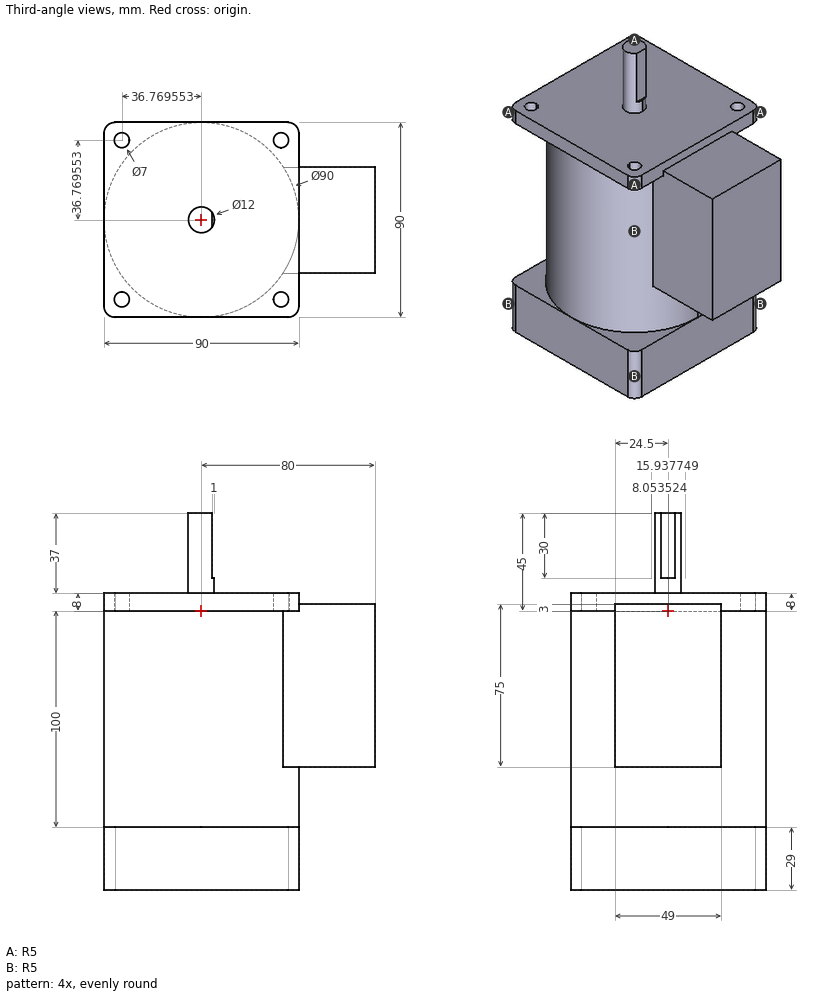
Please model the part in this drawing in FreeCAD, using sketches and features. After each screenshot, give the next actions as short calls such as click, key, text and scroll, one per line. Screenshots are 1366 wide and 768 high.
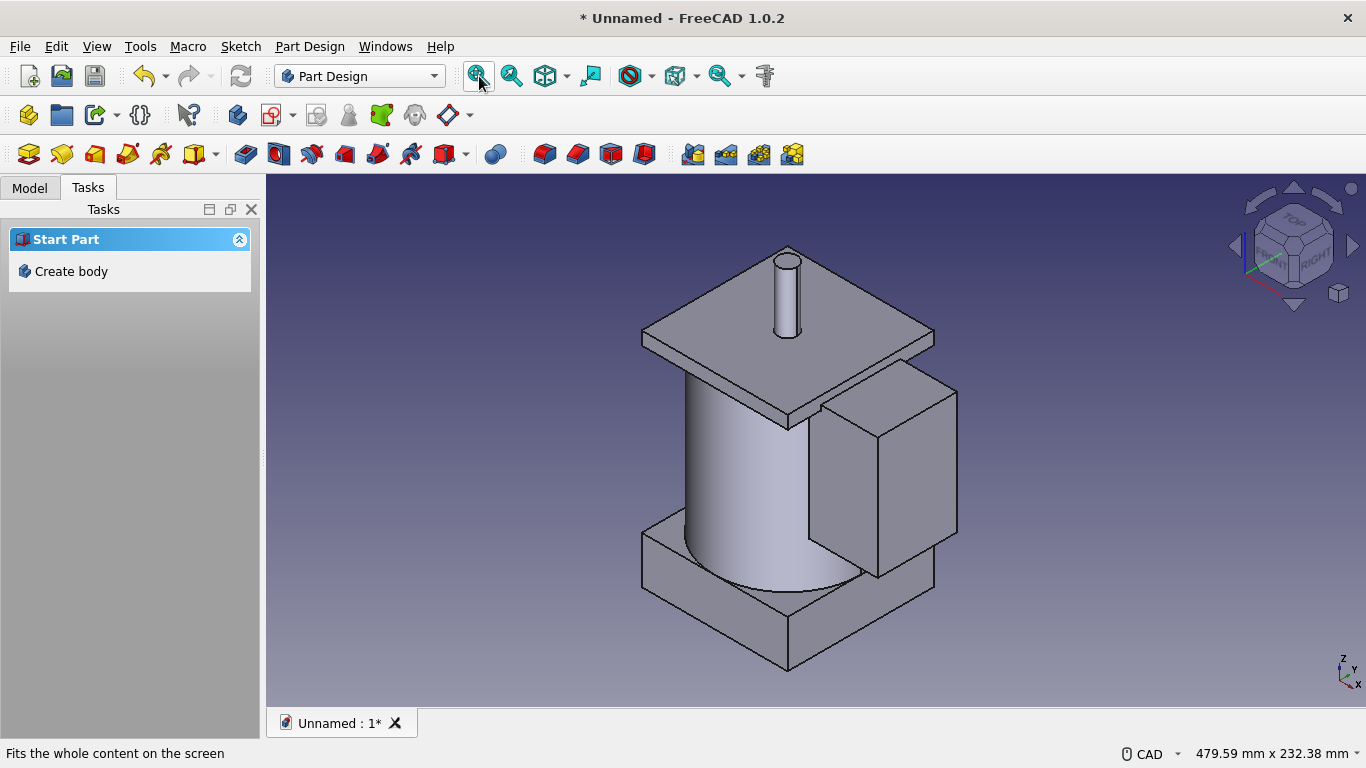
click(871, 329)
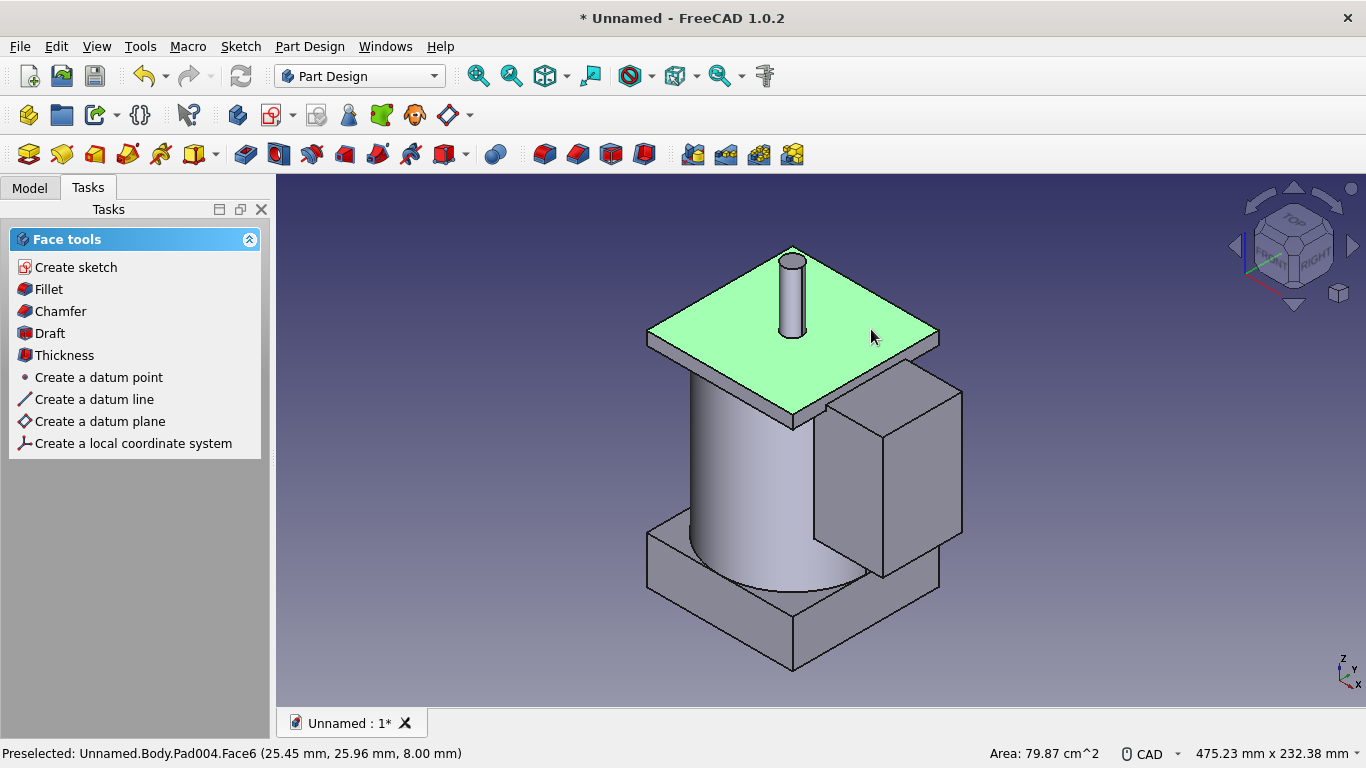
click(270, 116)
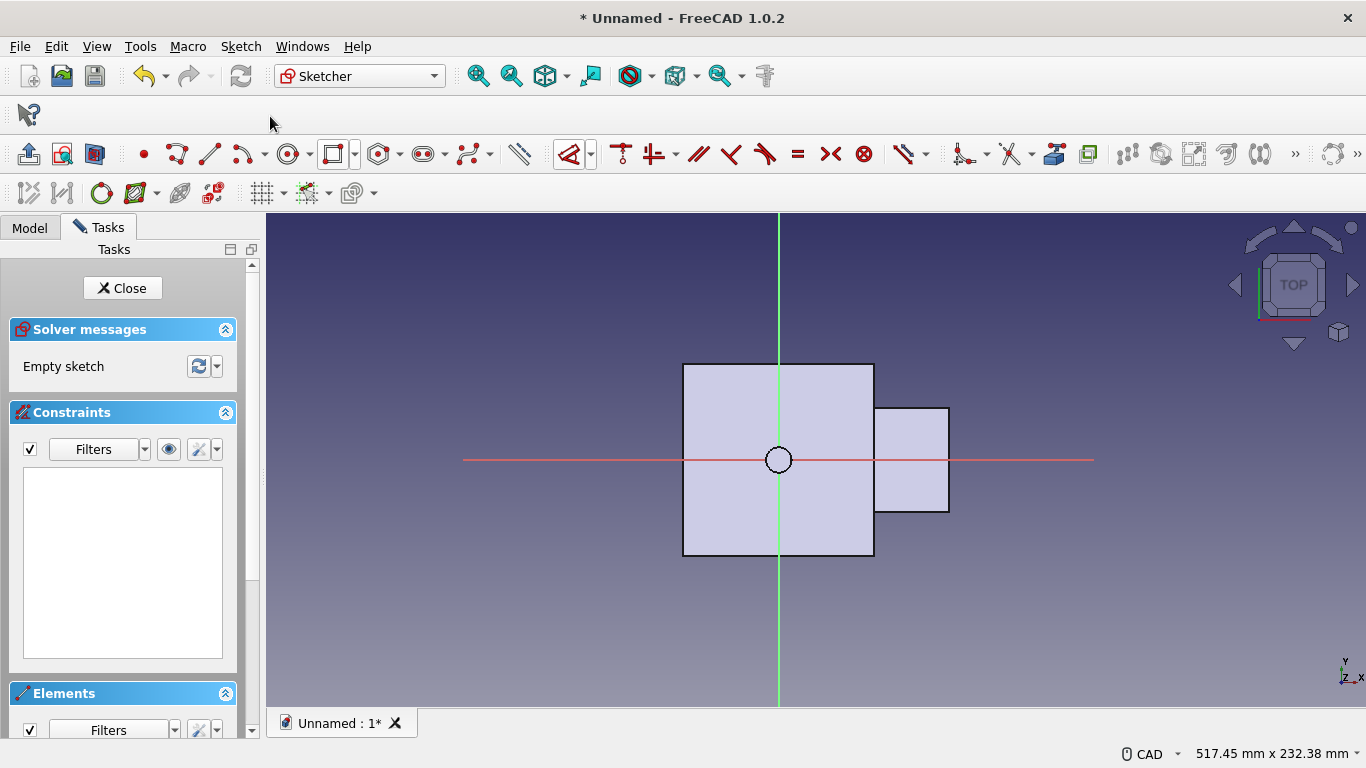
click(95, 154)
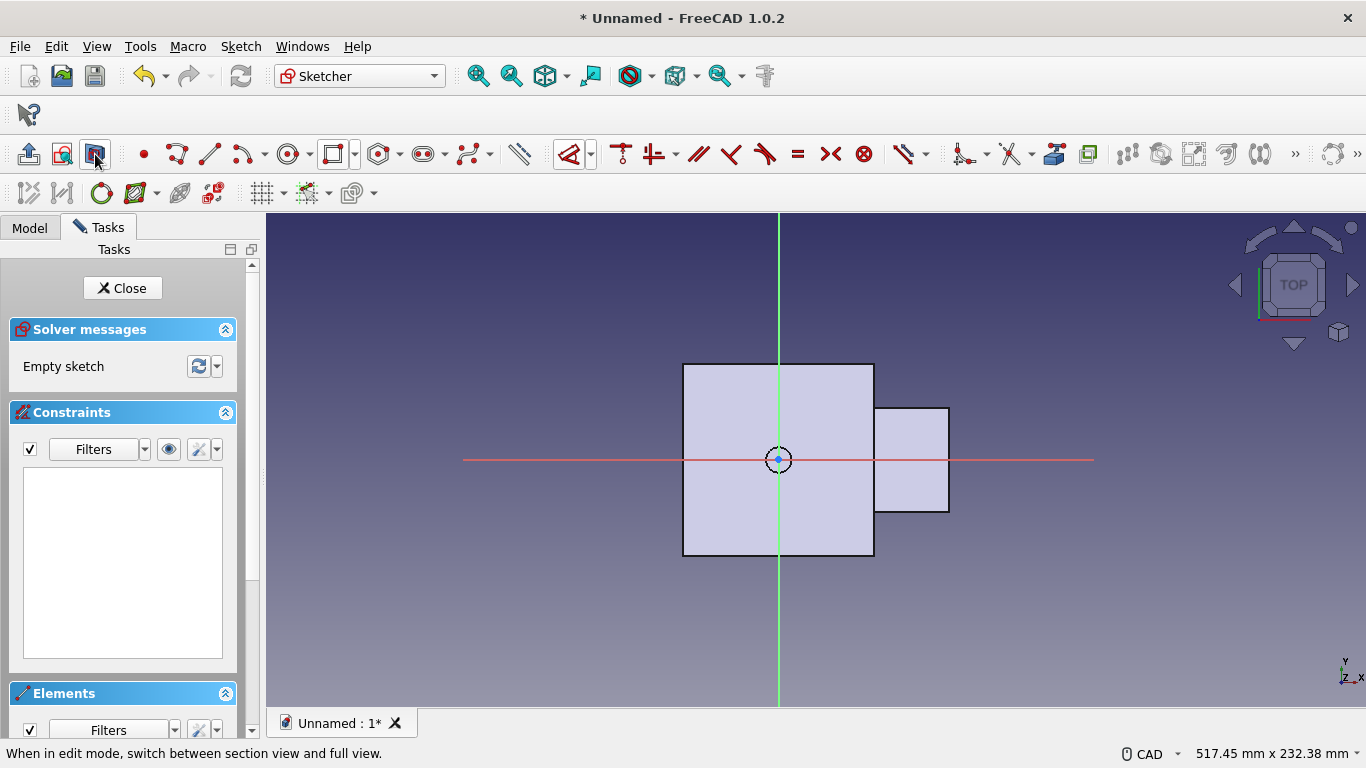
scroll(698, 378, up, 15)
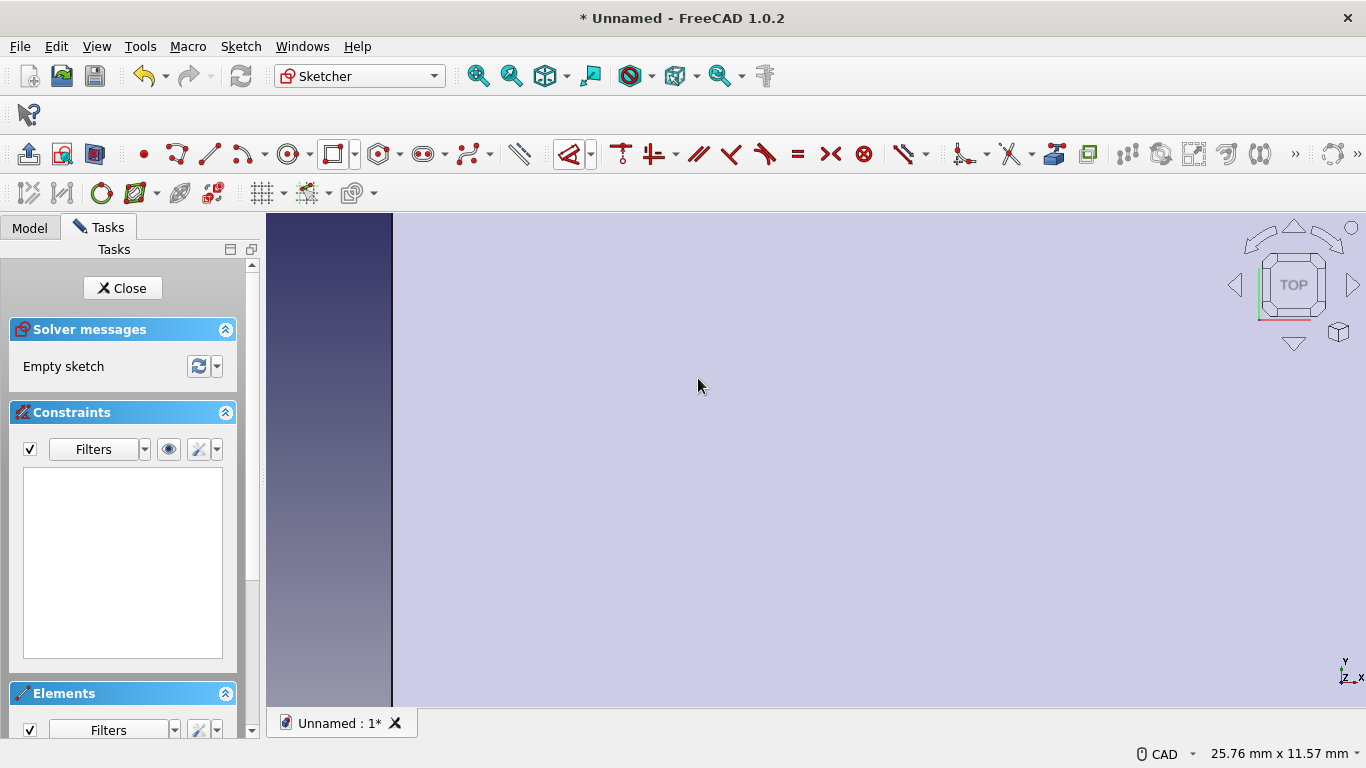
click(288, 154)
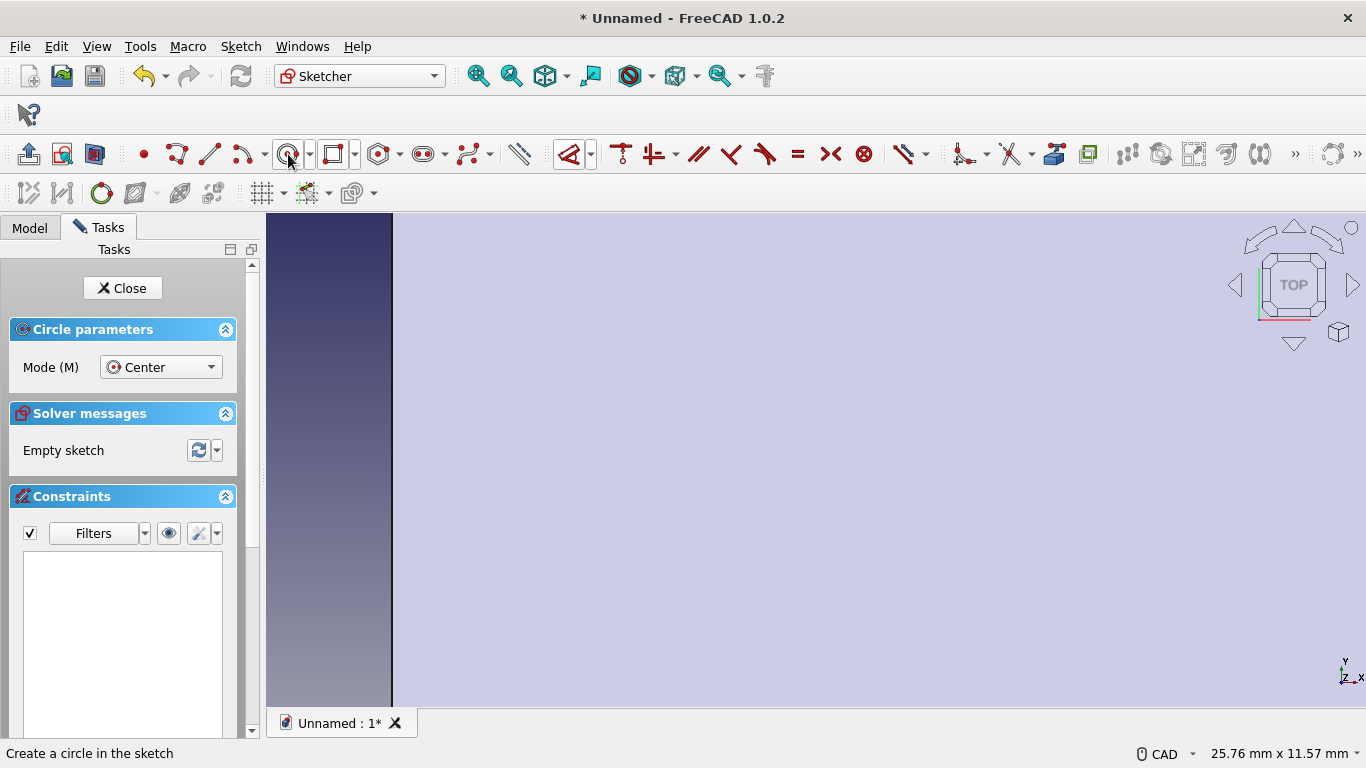
click(743, 449)
click(849, 343)
key(Escape)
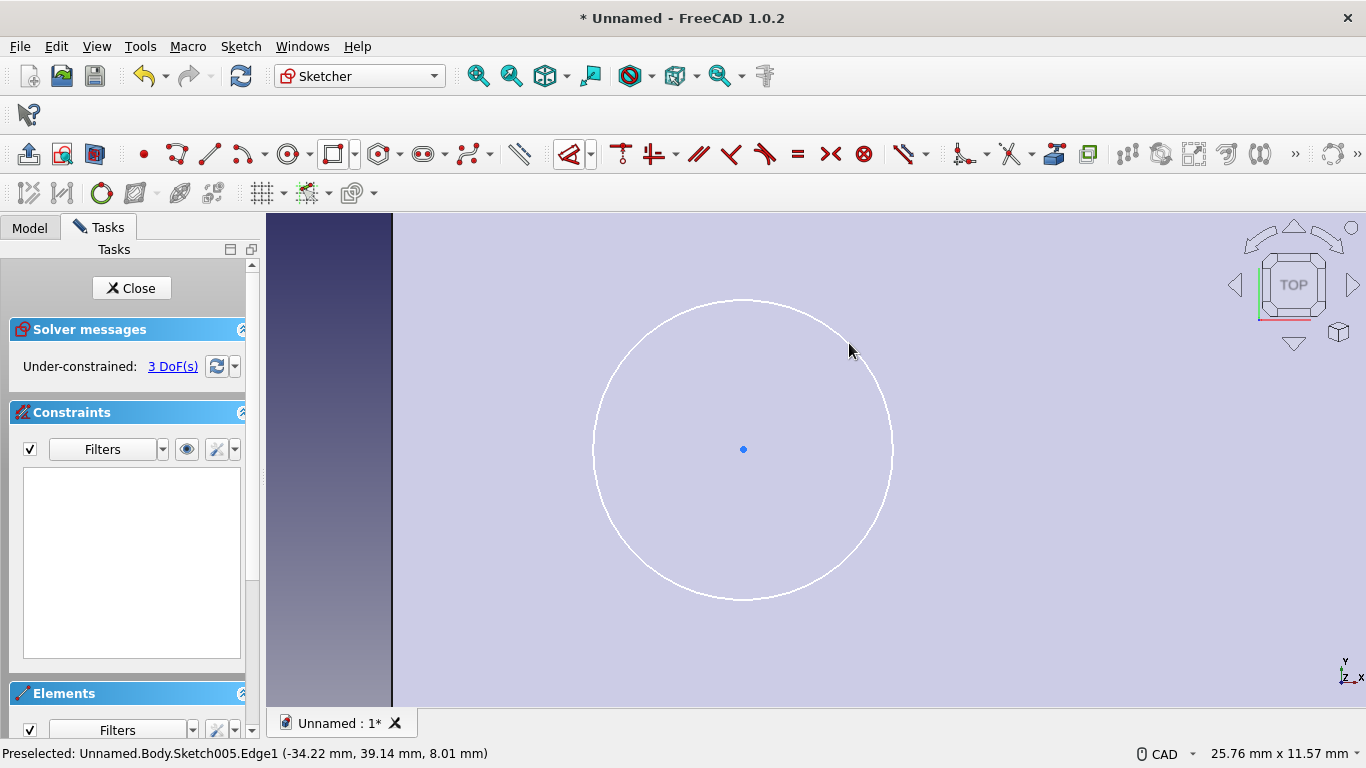
click(849, 344)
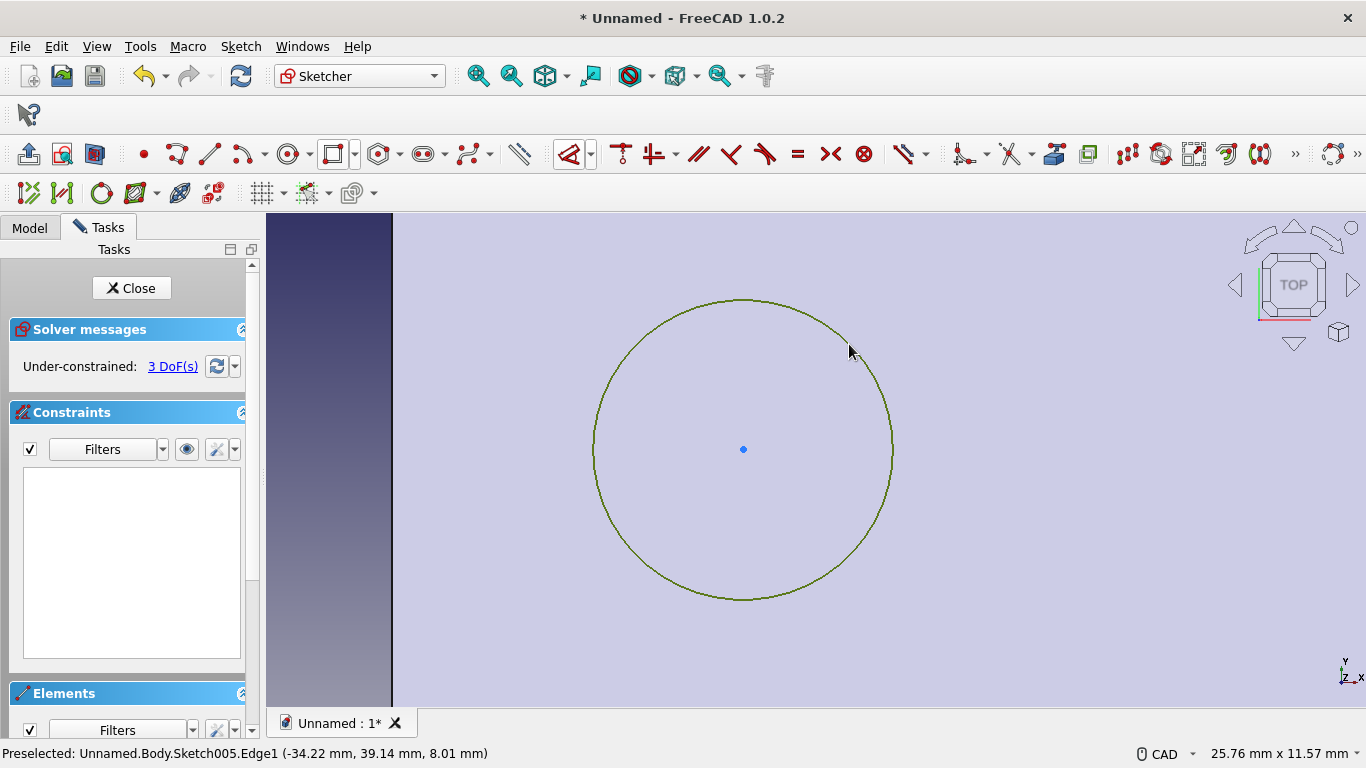
key(k)
key(o)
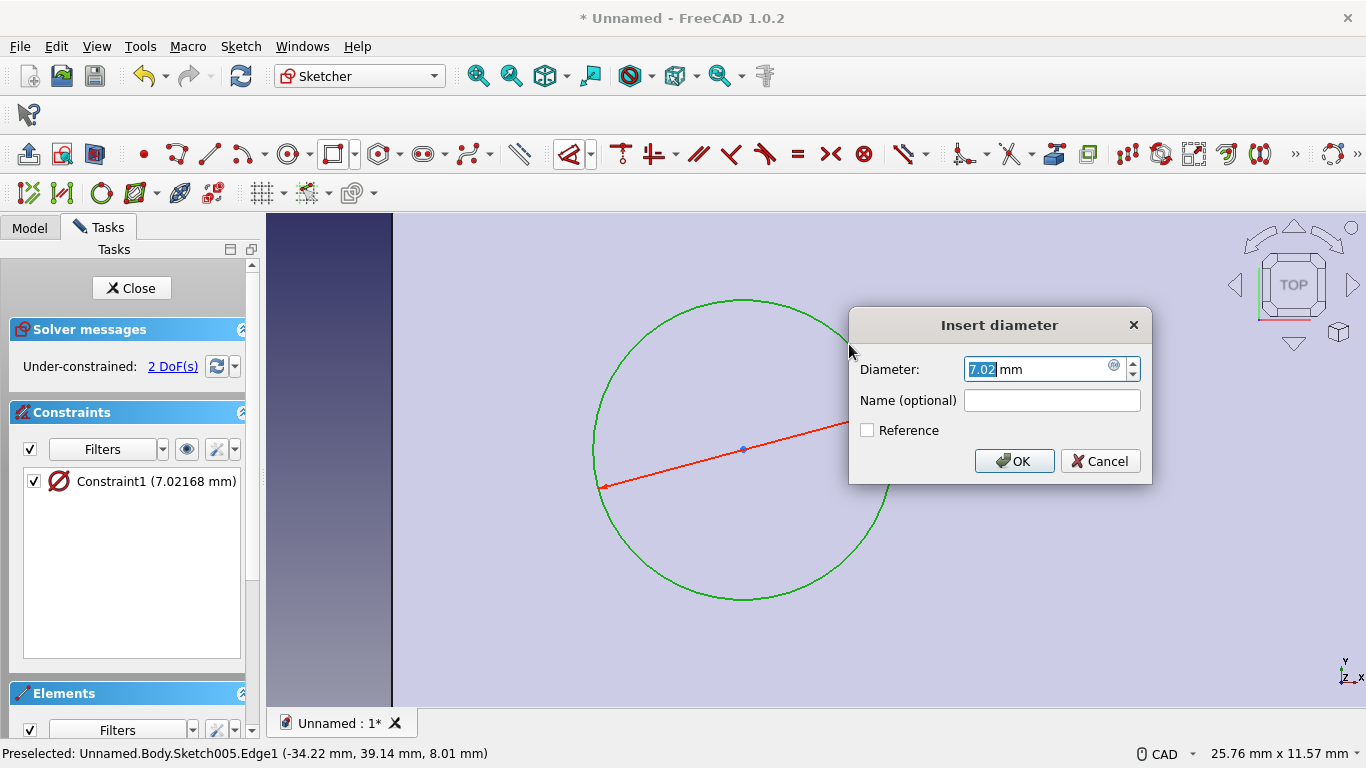
text(7)
key(Return)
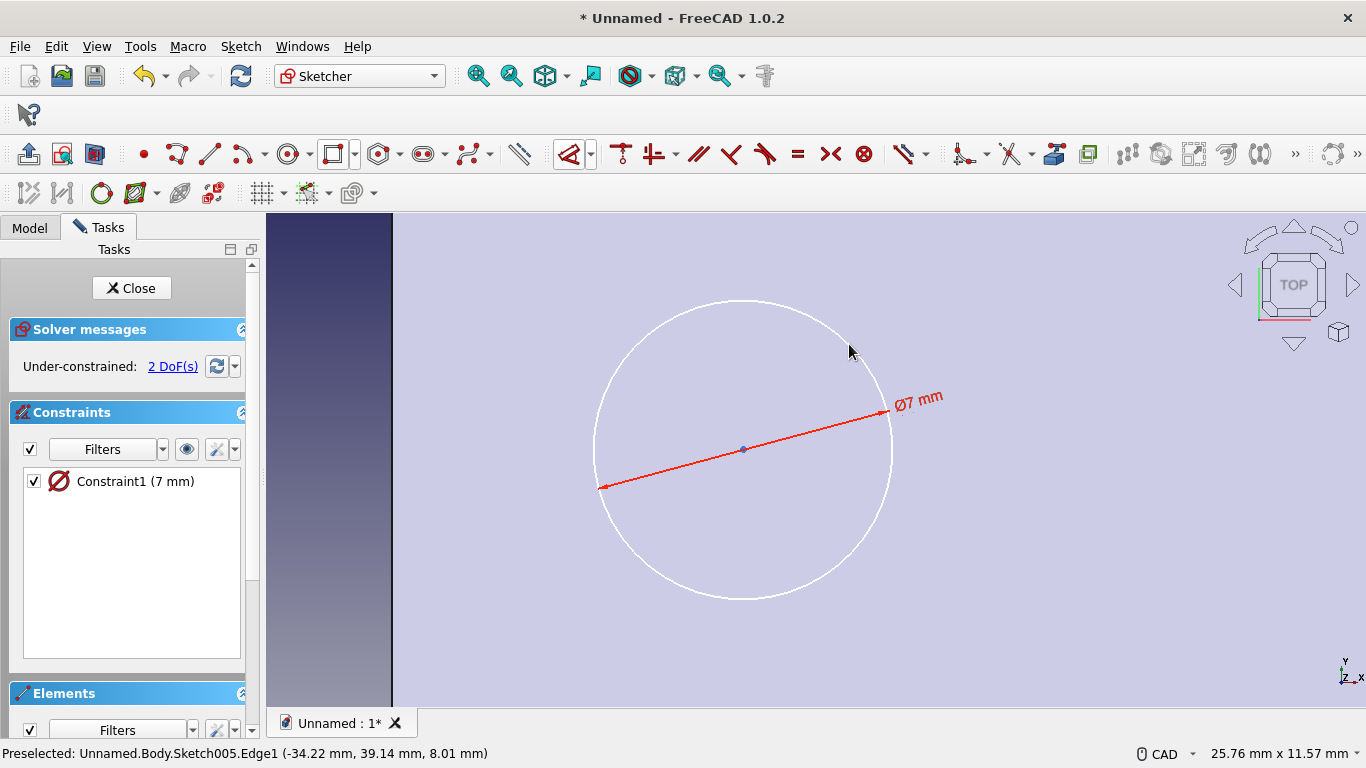
click(743, 450)